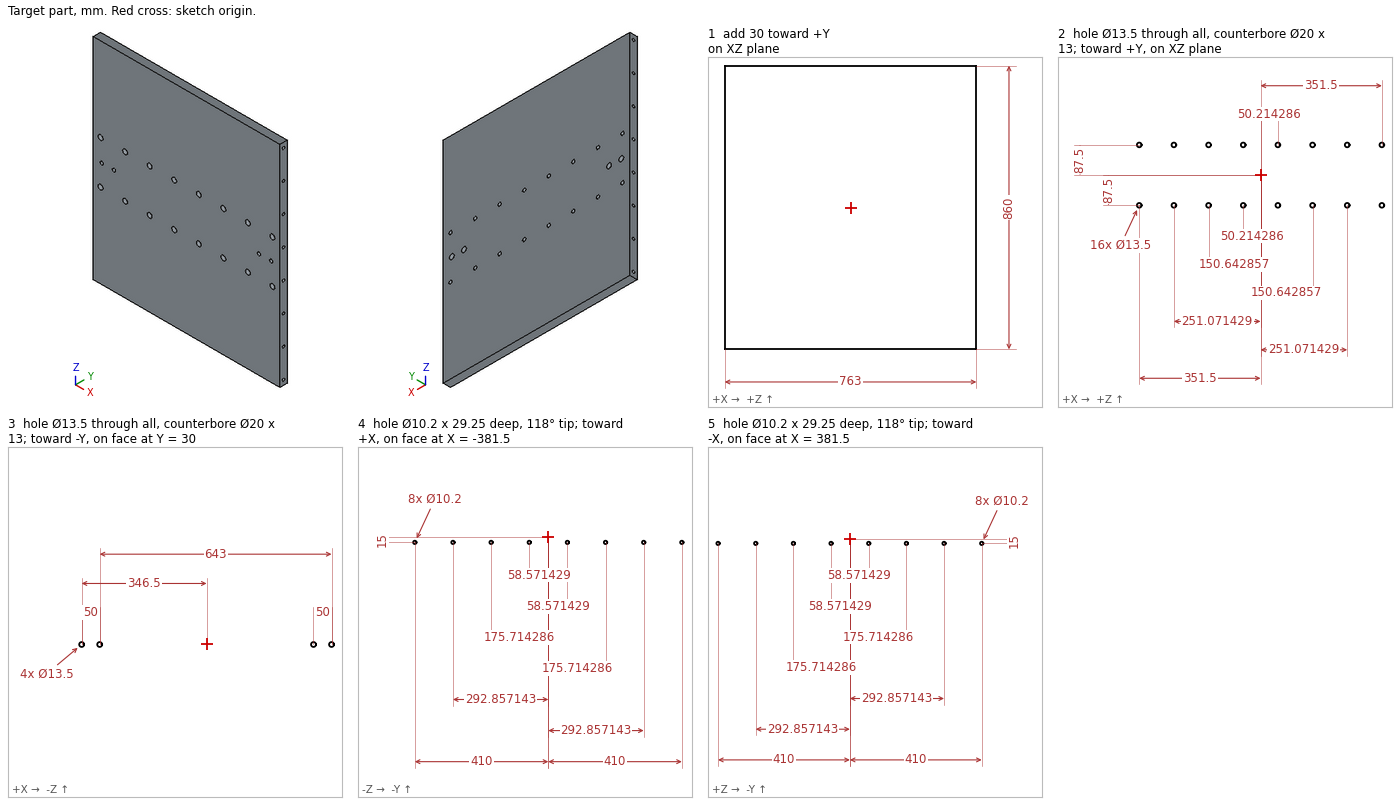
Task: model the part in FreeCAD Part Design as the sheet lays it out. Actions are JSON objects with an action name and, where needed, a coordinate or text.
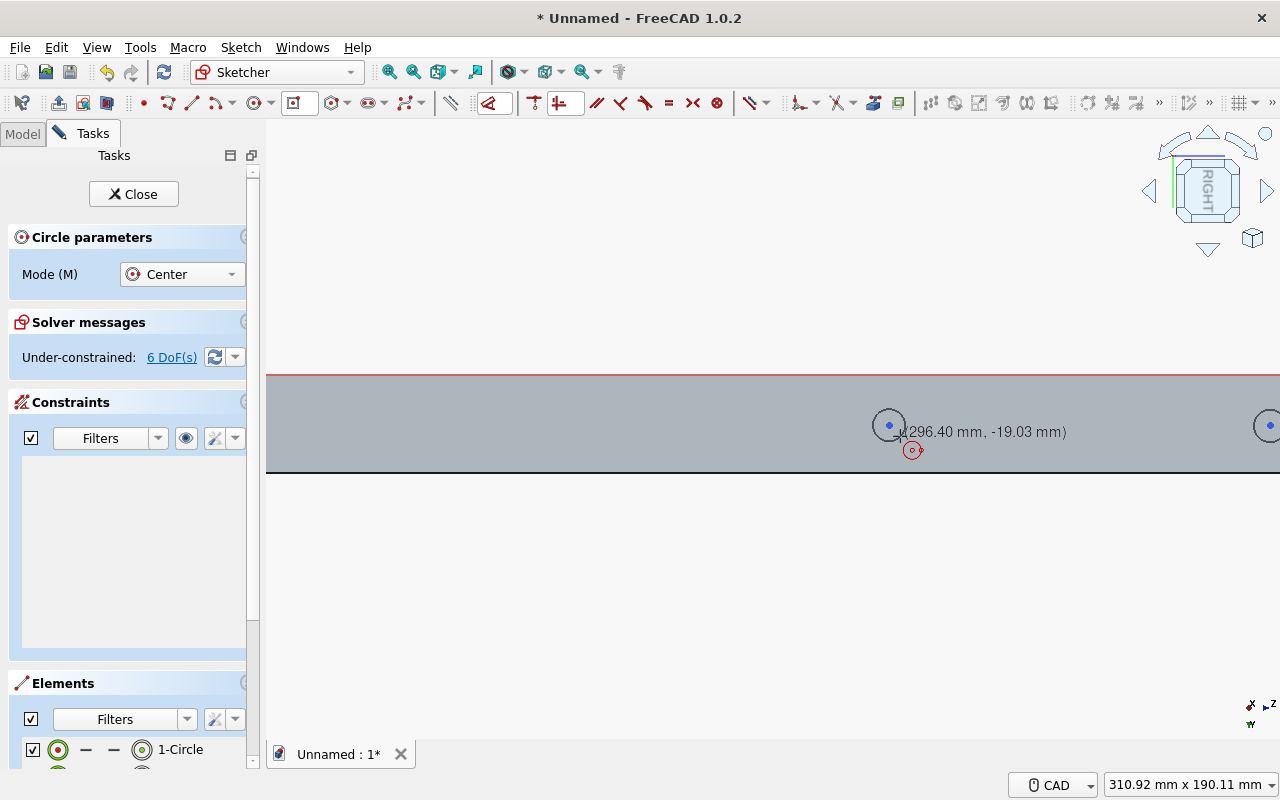
{"action": "scroll", "coordinate": [506, 424], "scroll_direction": "up", "scroll_amount": 2}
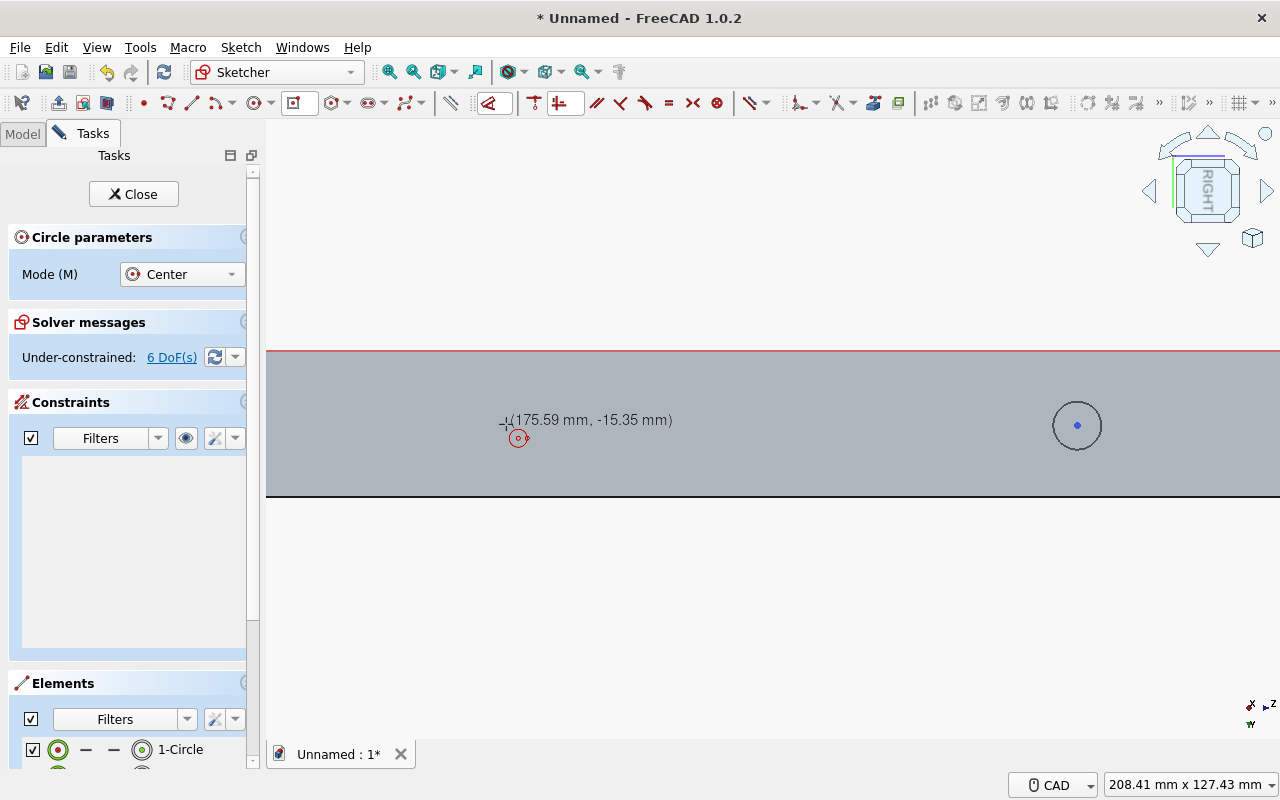
{"action": "scroll", "coordinate": [869, 434], "scroll_direction": "down", "scroll_amount": 10}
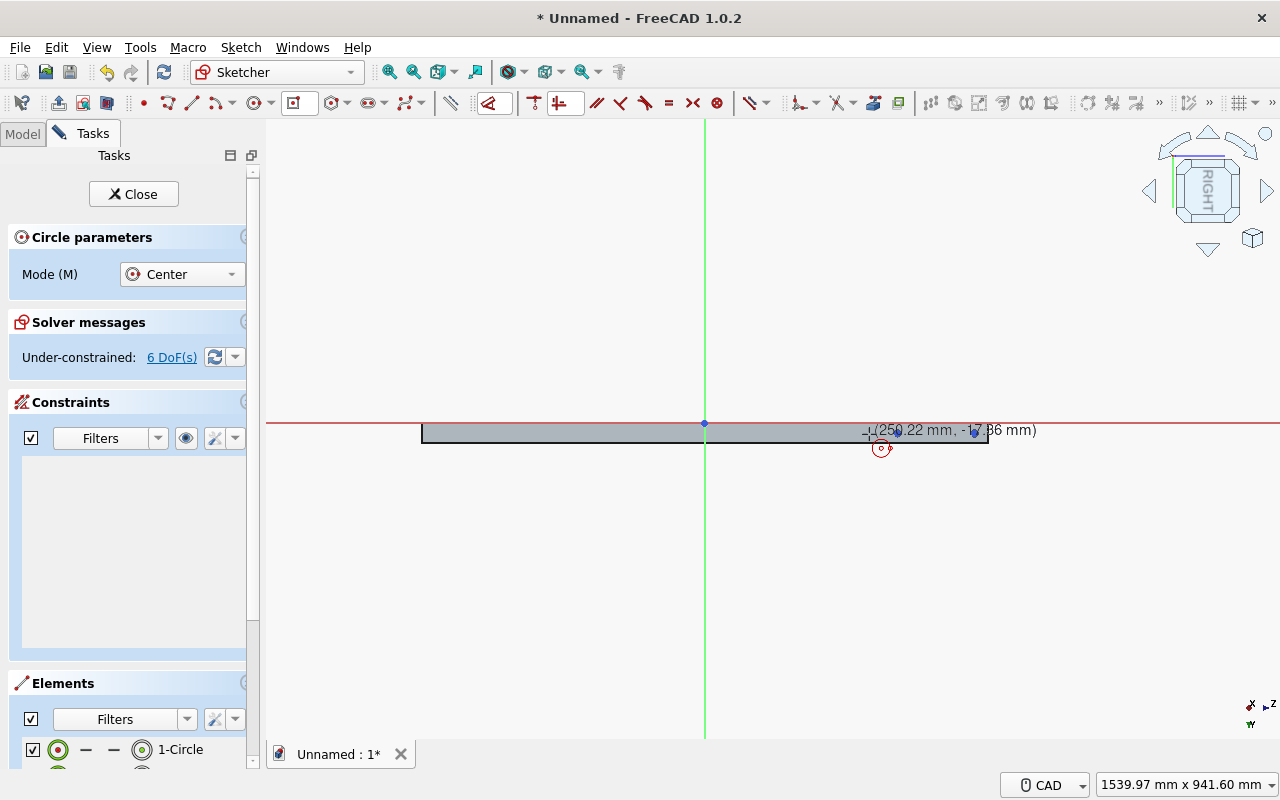
{"action": "scroll", "coordinate": [820, 433], "scroll_direction": "up", "scroll_amount": 3}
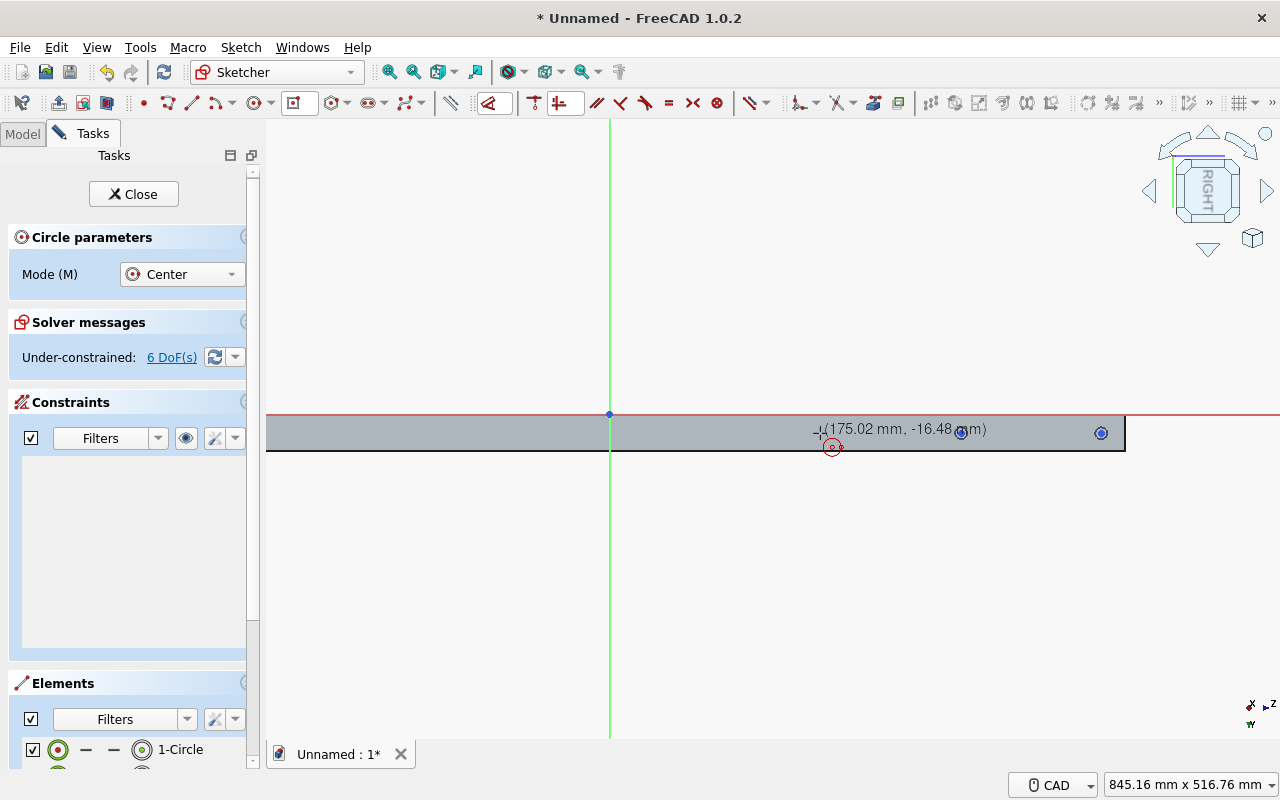
{"action": "left_click", "coordinate": [820, 433]}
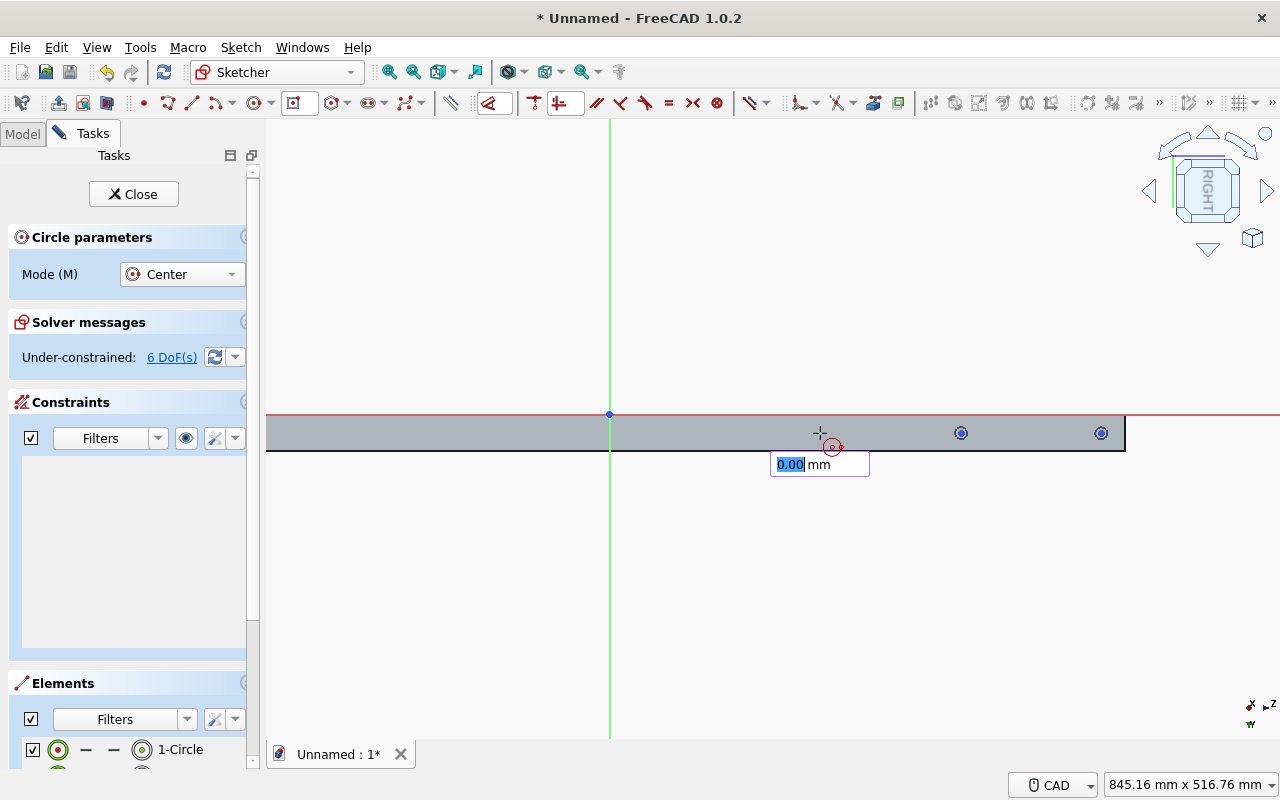
{"action": "scroll", "coordinate": [825, 437], "scroll_direction": "up", "scroll_amount": 5}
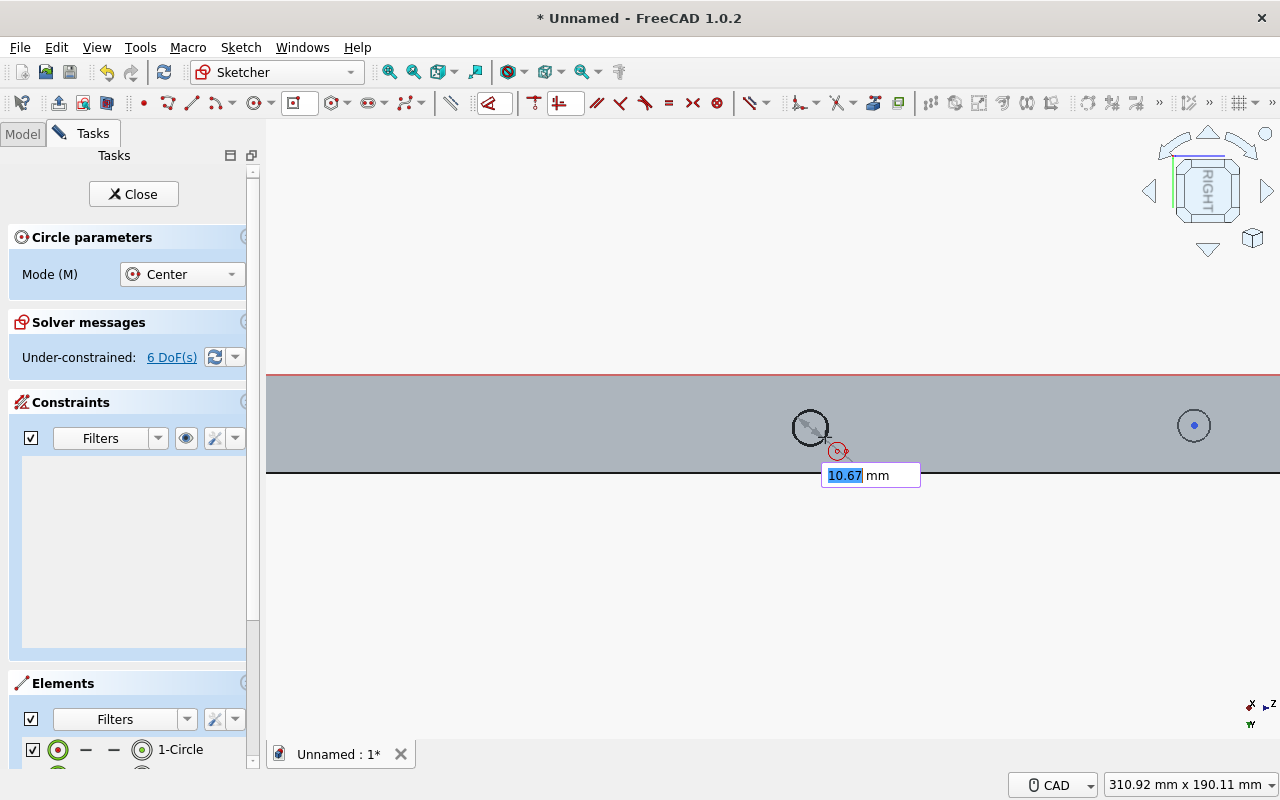
{"action": "left_click", "coordinate": [823, 436]}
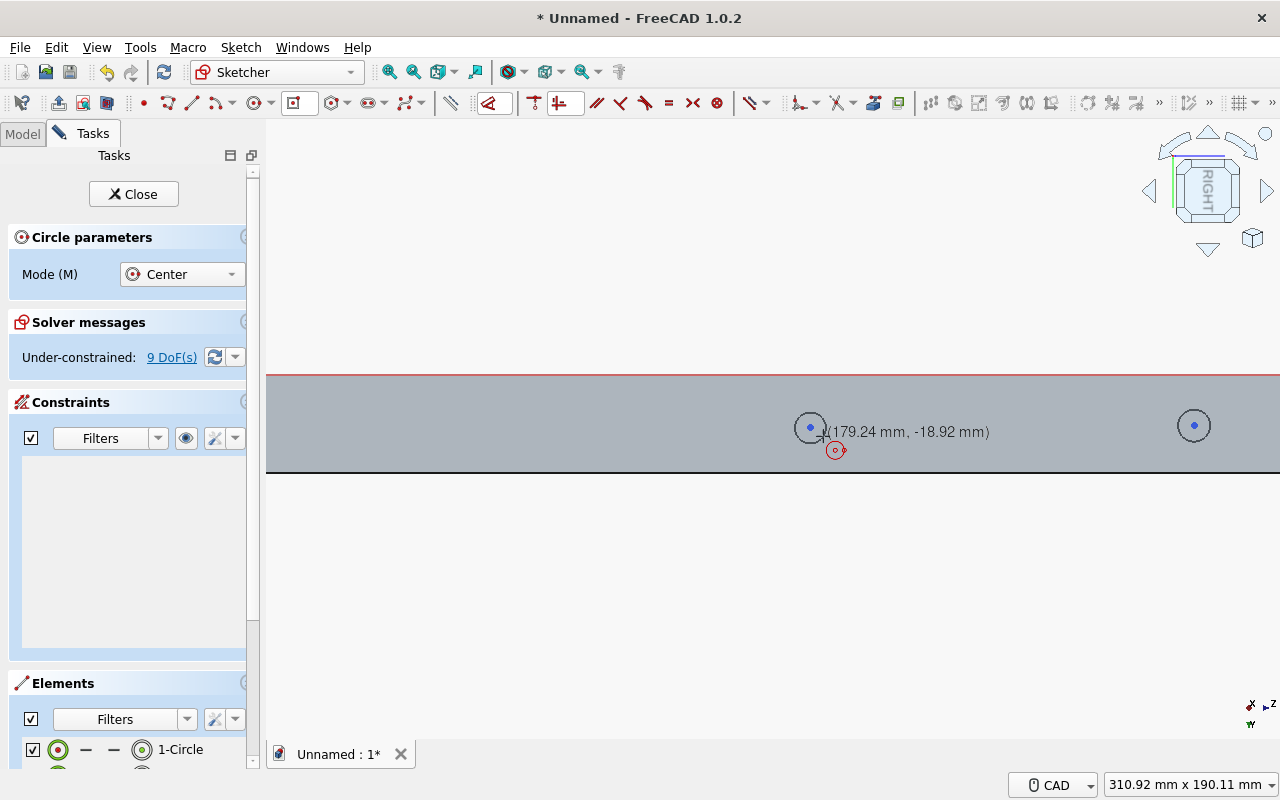
{"action": "scroll", "coordinate": [429, 424], "scroll_direction": "up", "scroll_amount": 2}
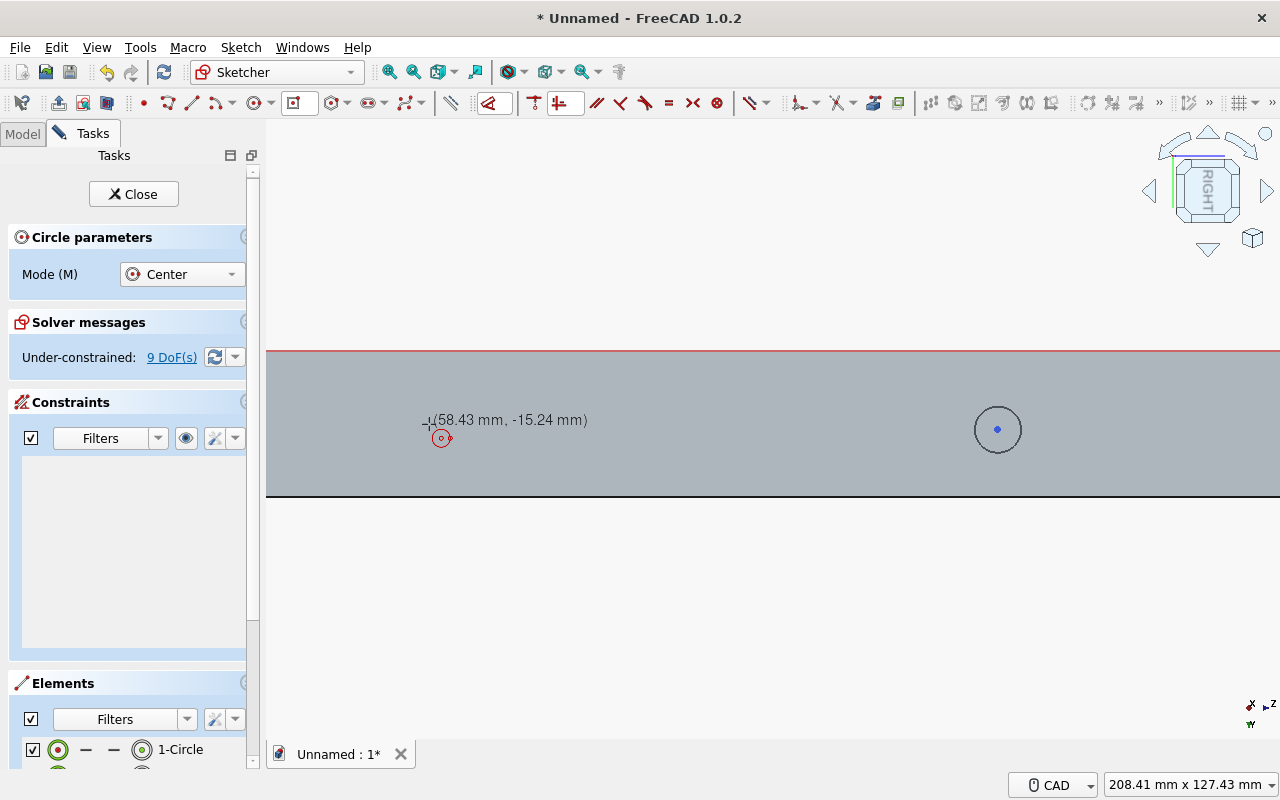
{"action": "scroll", "coordinate": [792, 434], "scroll_direction": "down", "scroll_amount": 10}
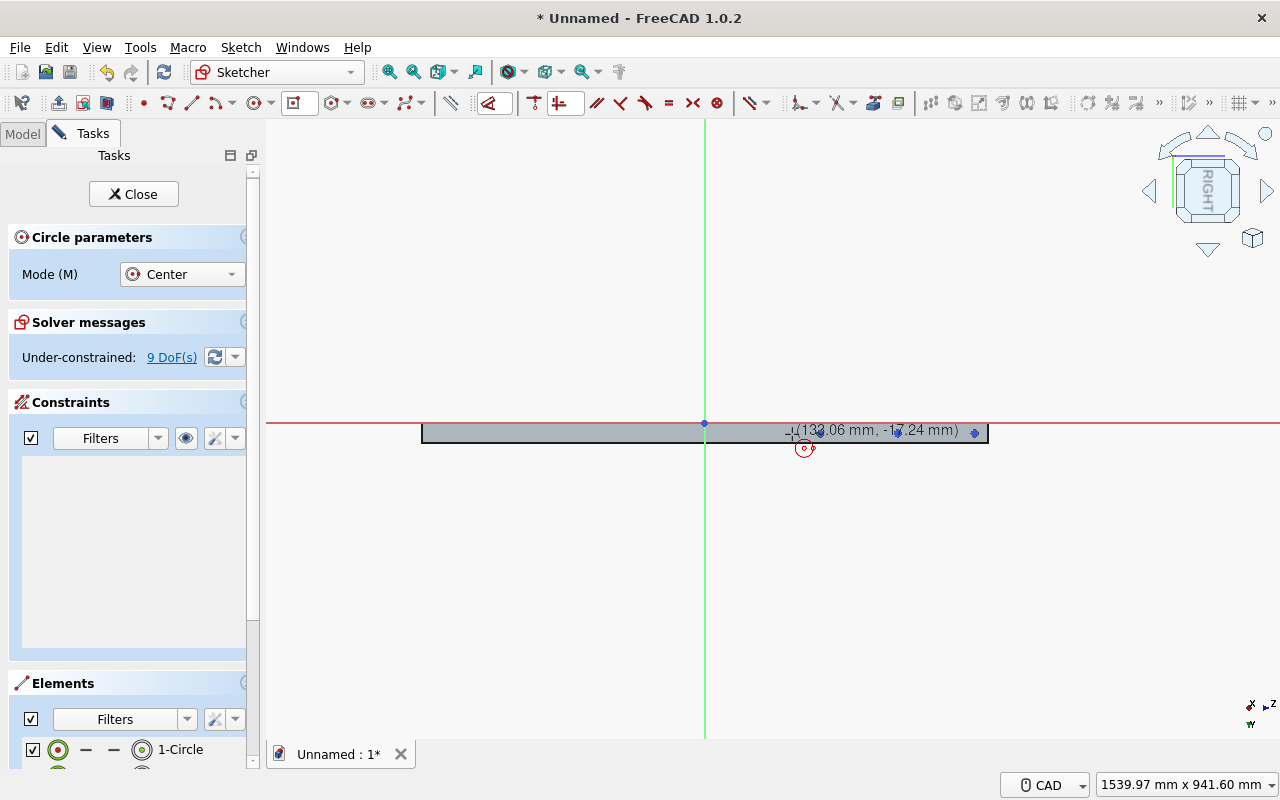
{"action": "scroll", "coordinate": [743, 433], "scroll_direction": "up", "scroll_amount": 3}